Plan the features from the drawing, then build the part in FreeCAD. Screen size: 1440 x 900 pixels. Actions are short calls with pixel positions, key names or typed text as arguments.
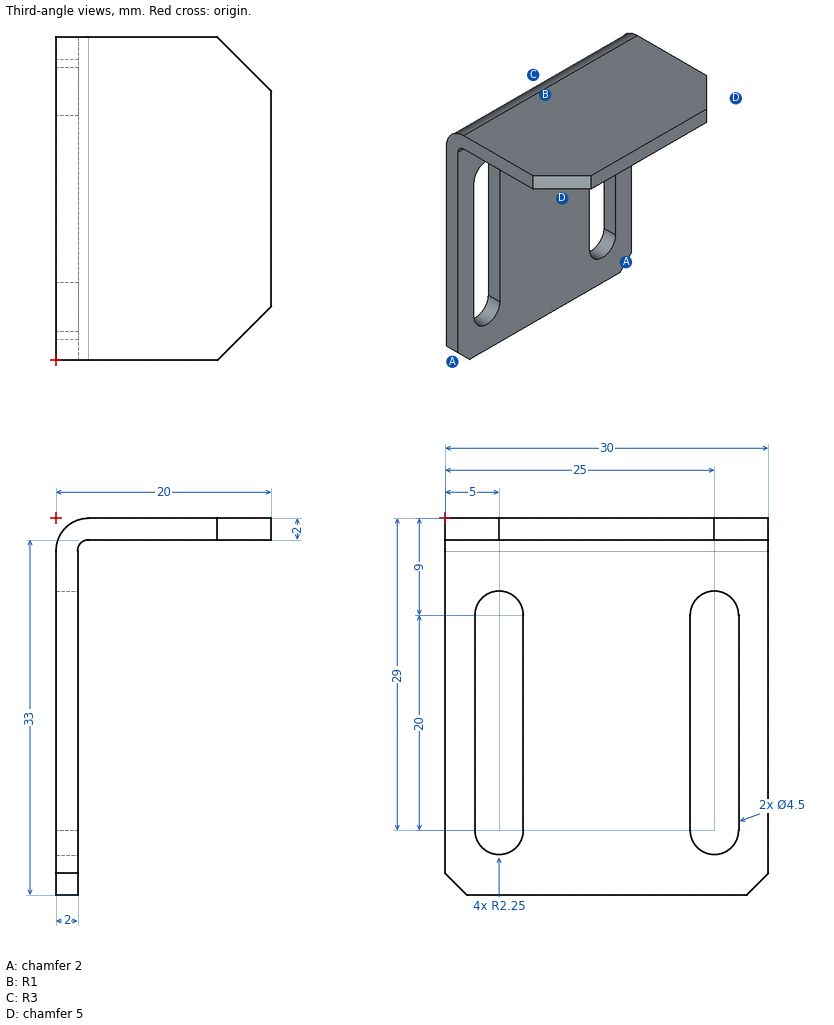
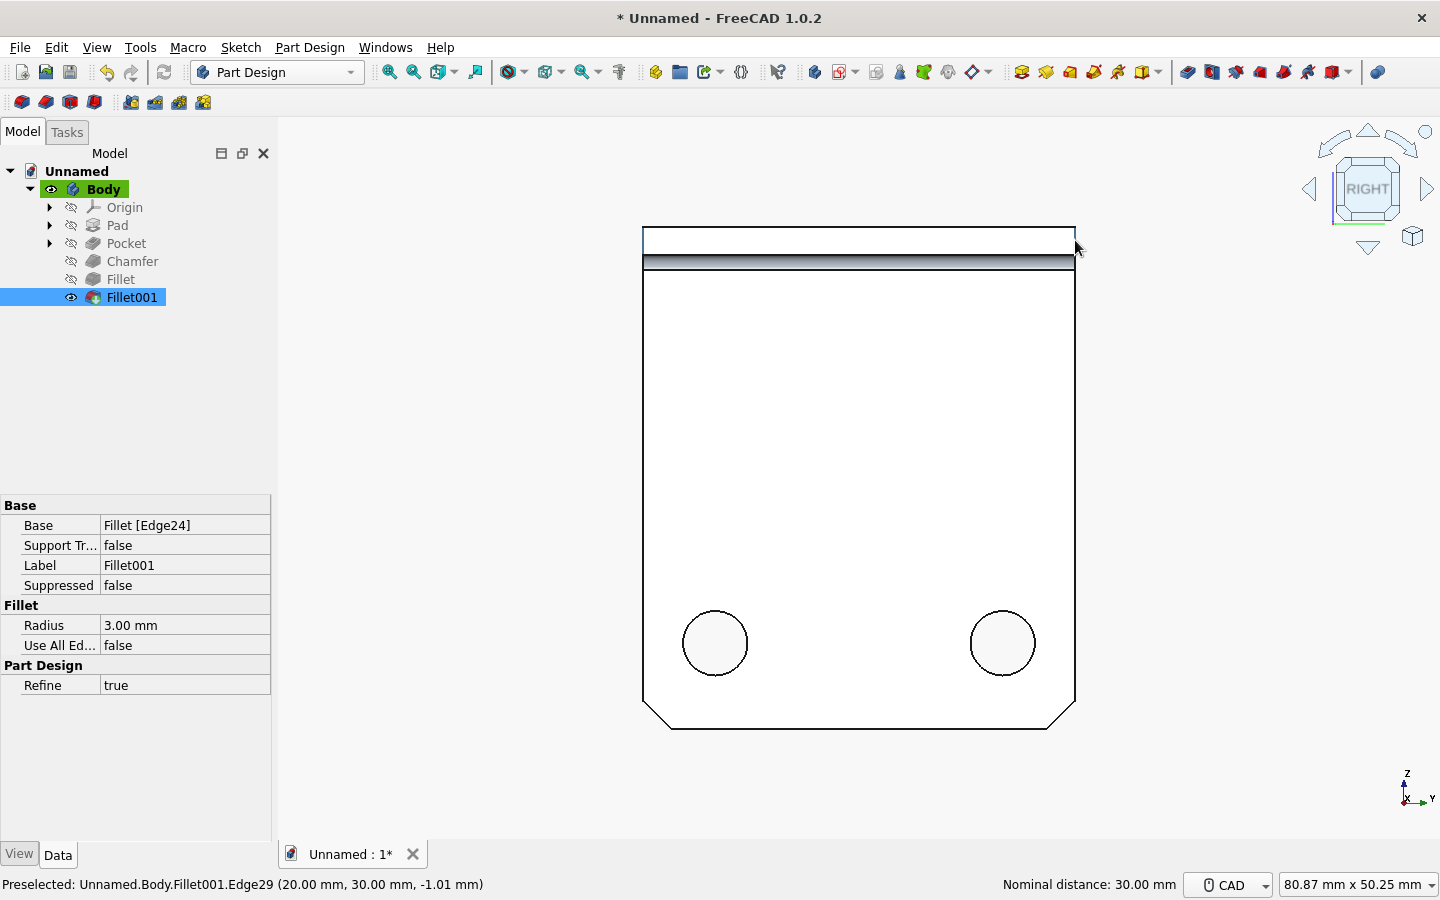
click(46, 102)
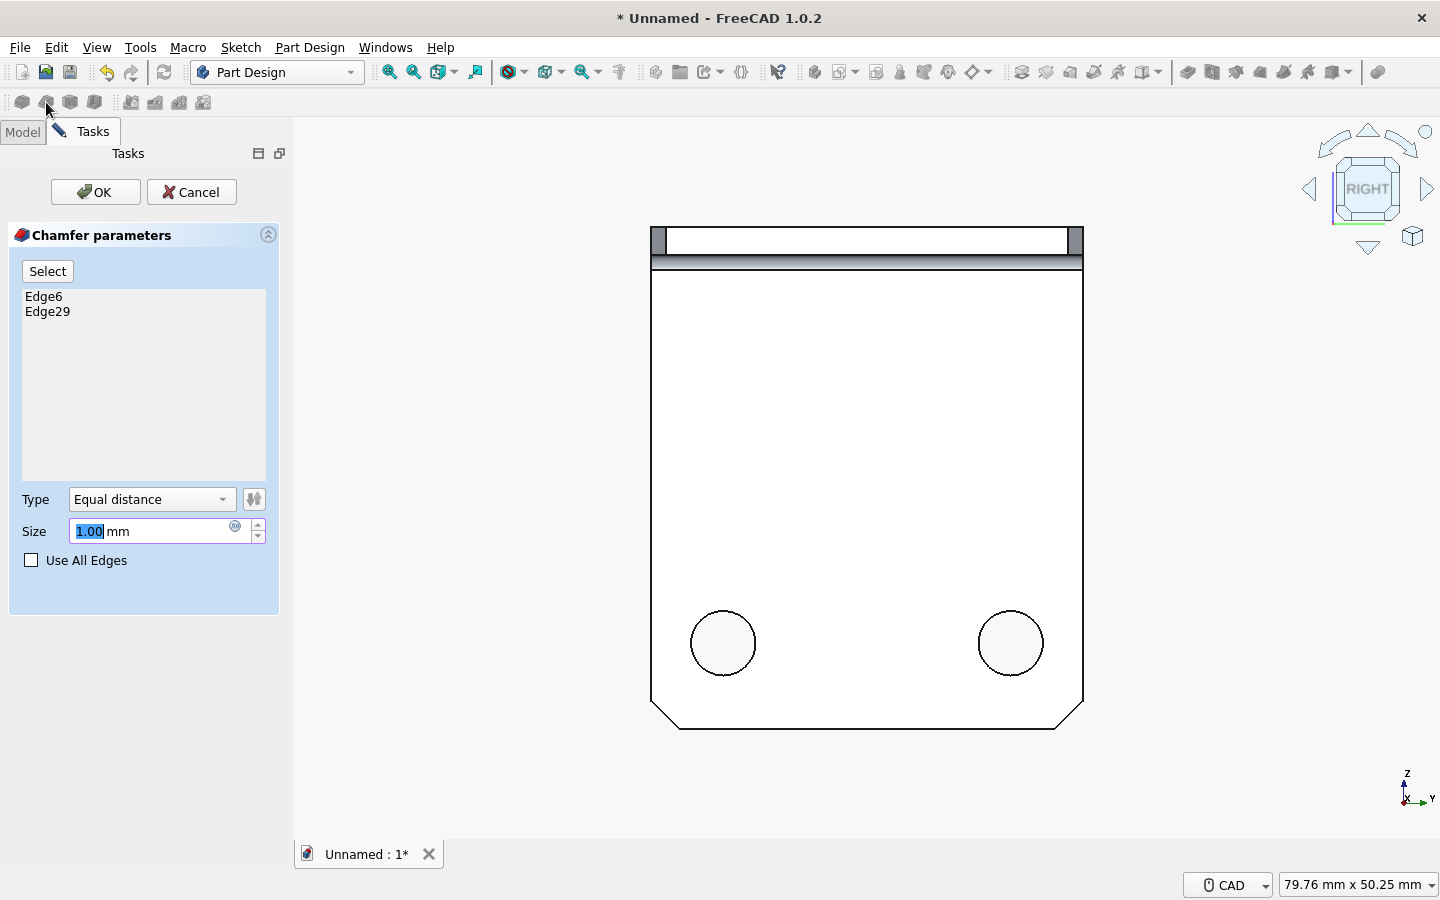
text(5)
key(Tab)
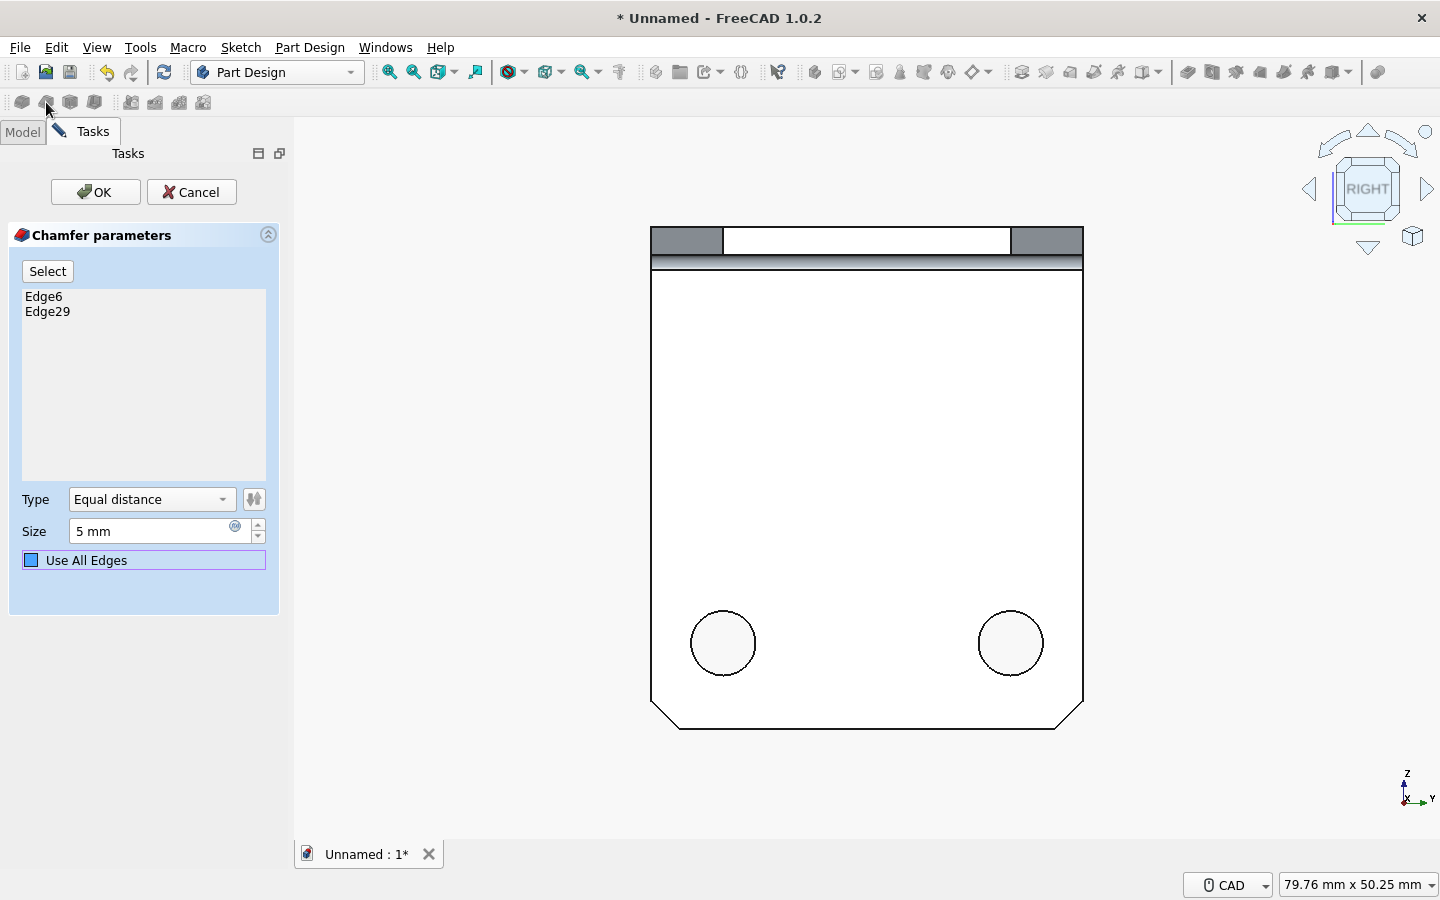
click(96, 192)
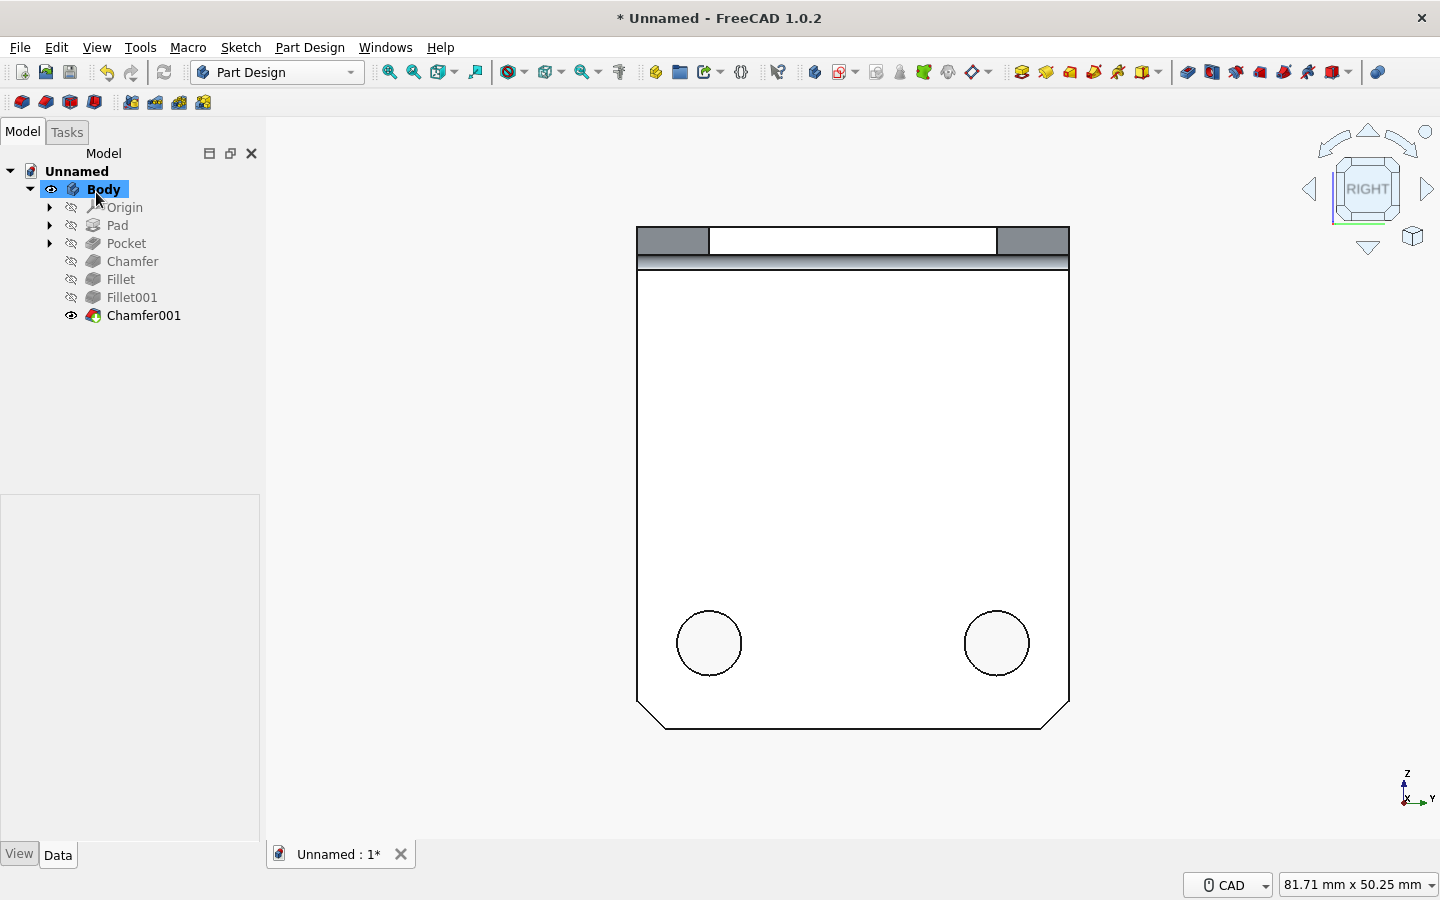
click(853, 499)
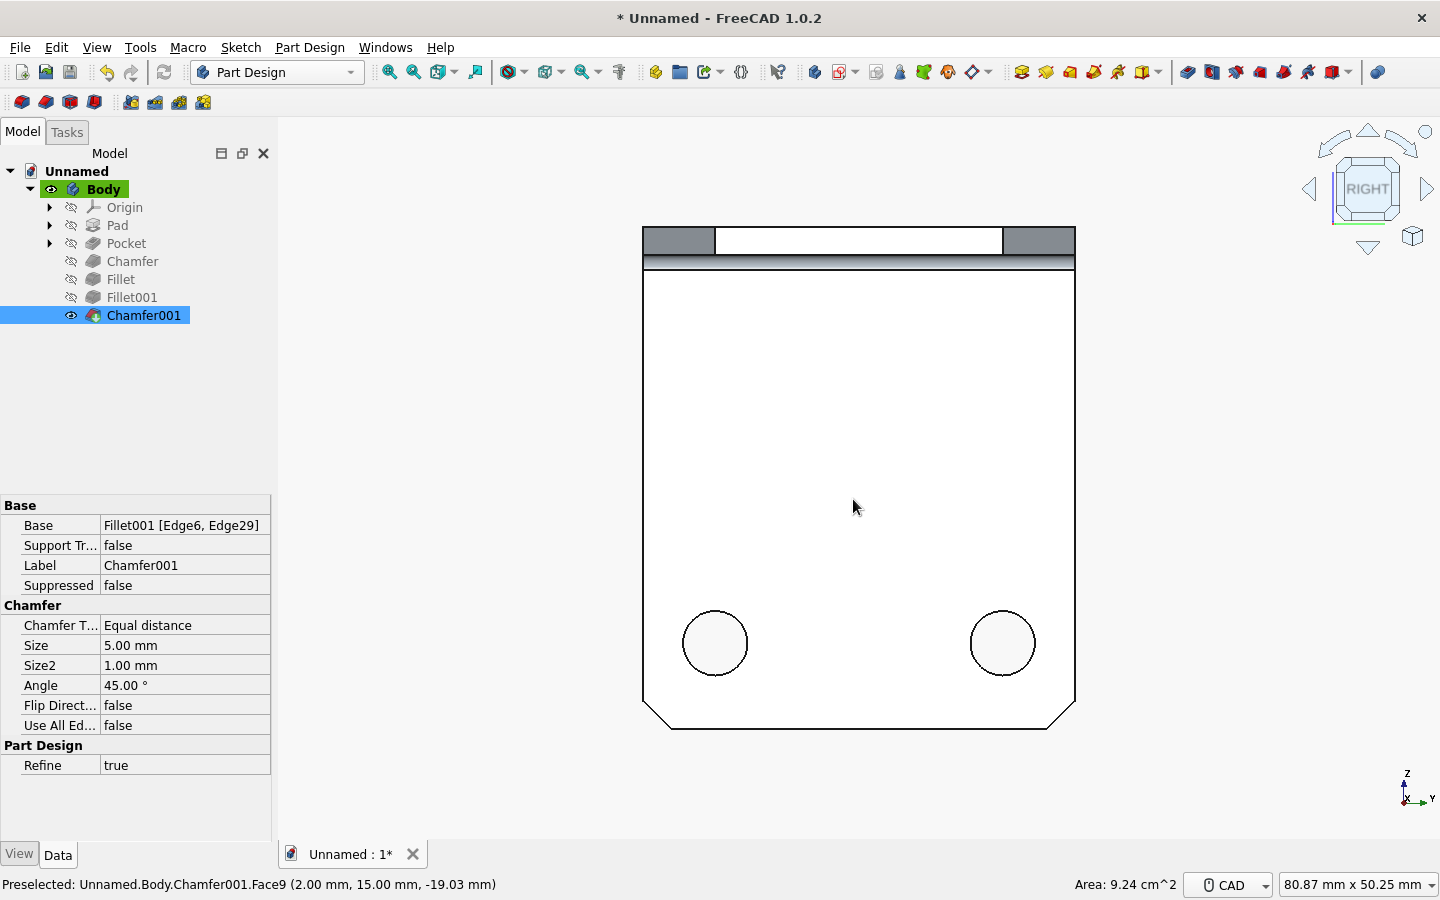
click(840, 72)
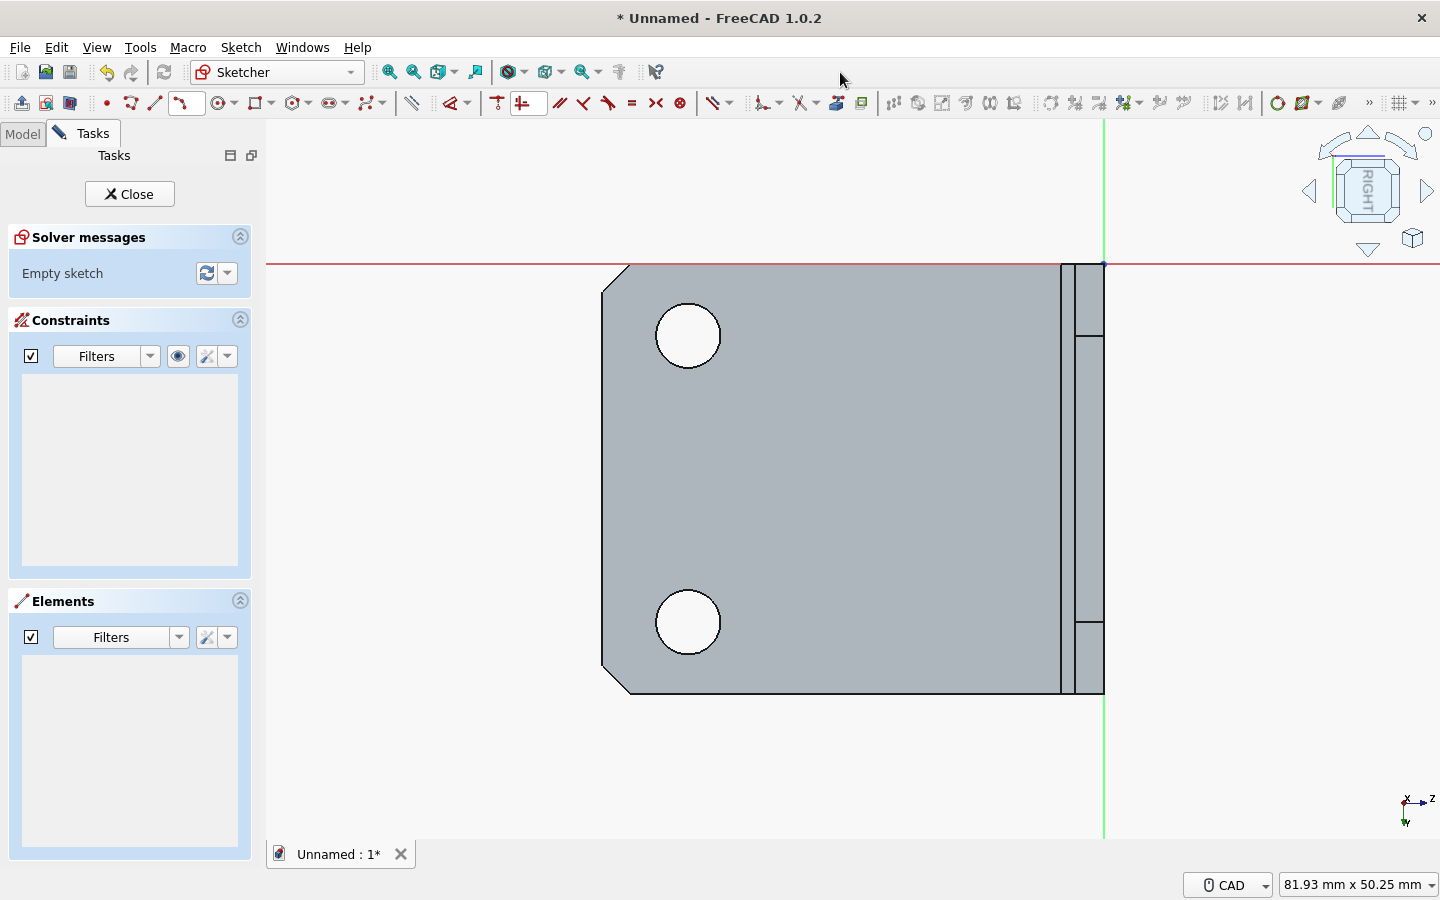
click(330, 104)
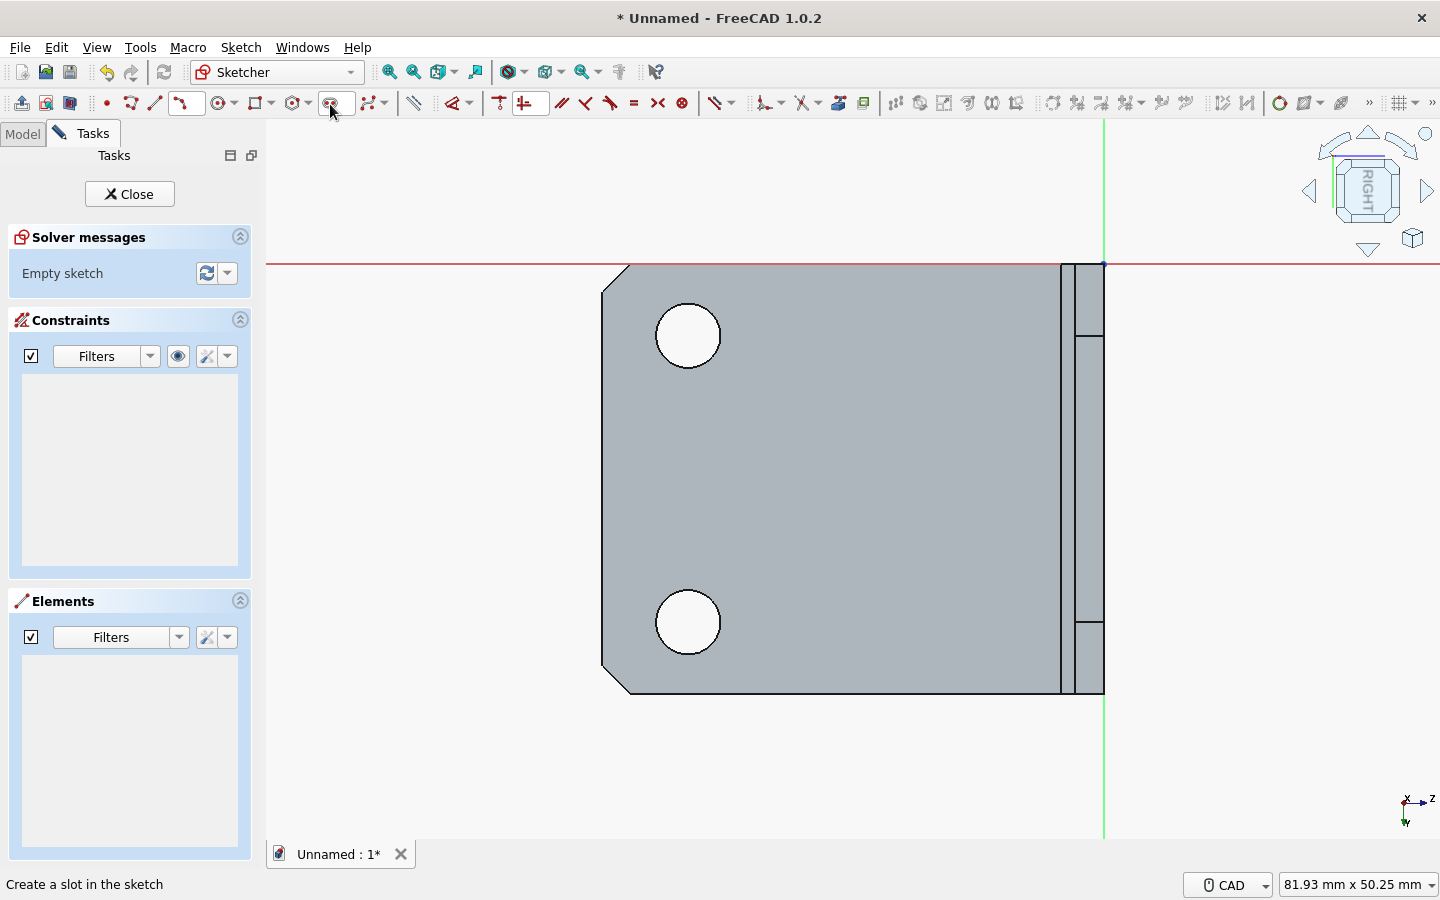
click(688, 336)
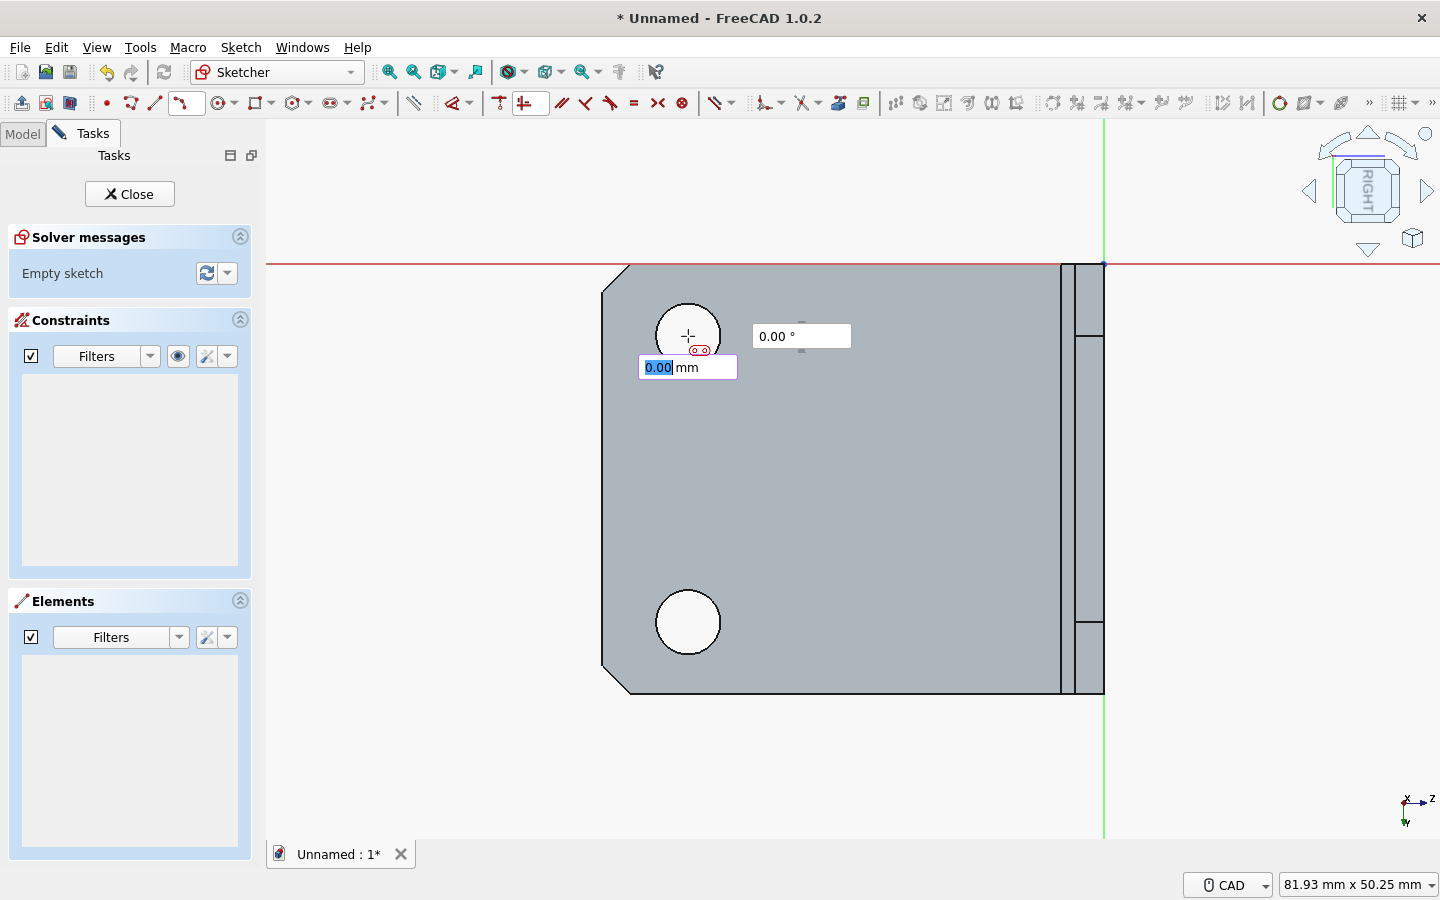
click(975, 336)